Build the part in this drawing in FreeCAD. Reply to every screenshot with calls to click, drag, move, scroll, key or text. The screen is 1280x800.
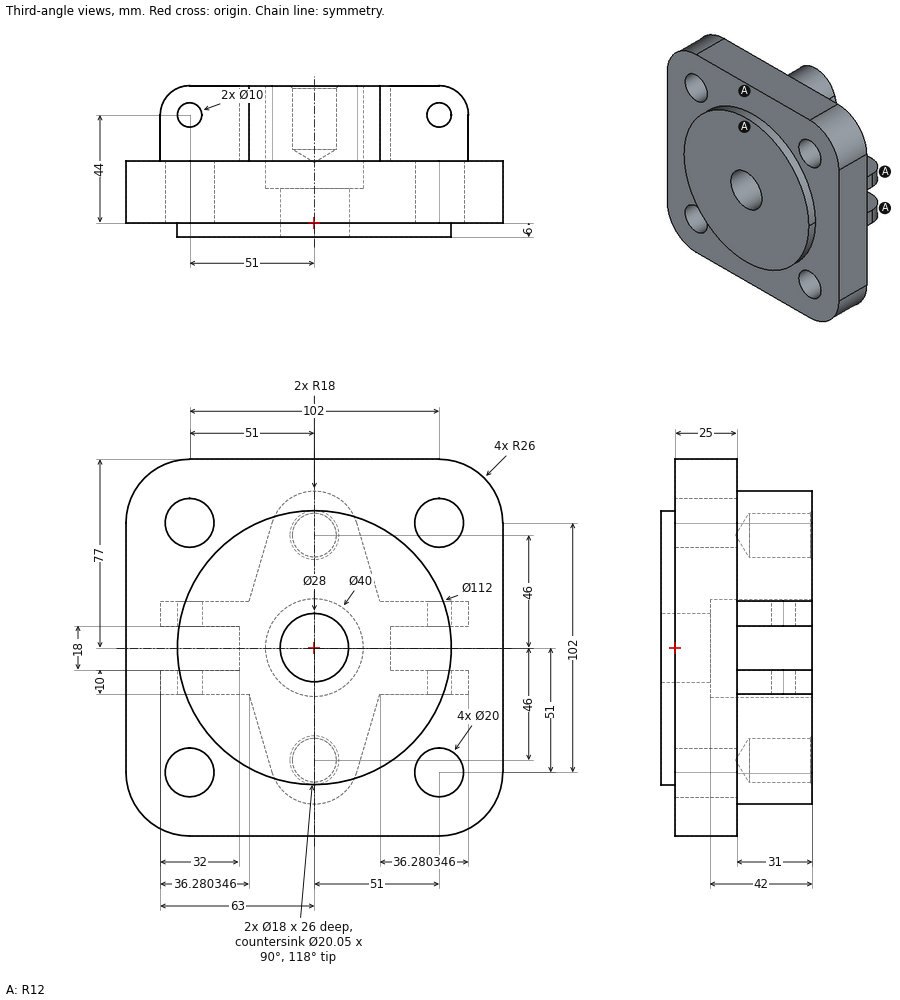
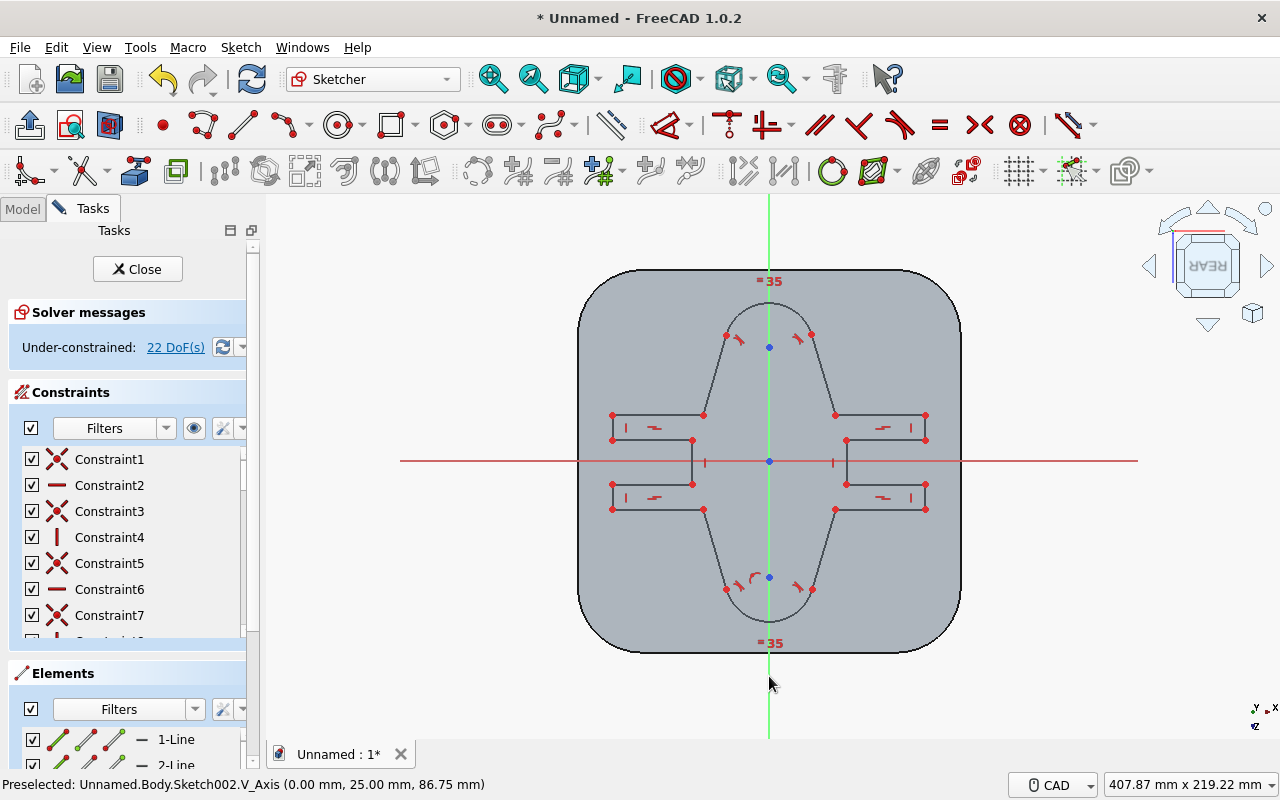
click(769, 348)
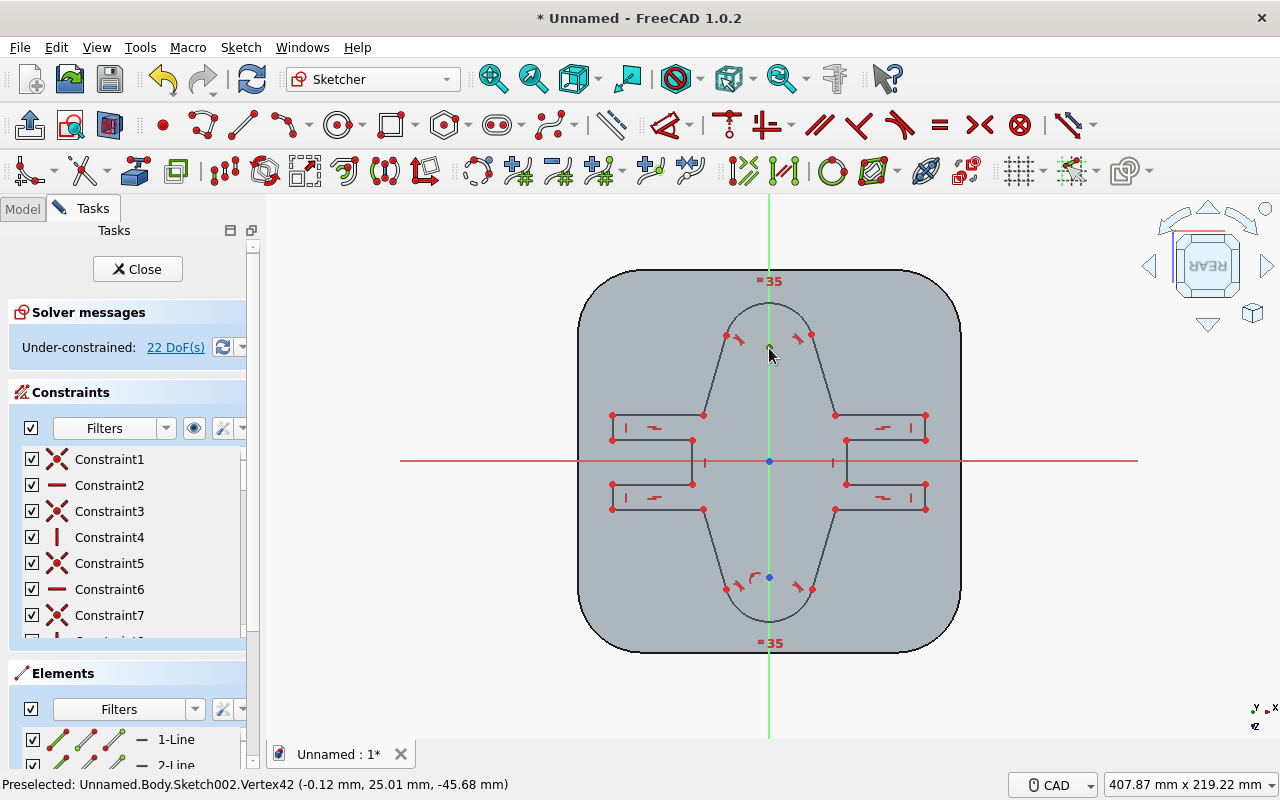
click(769, 676)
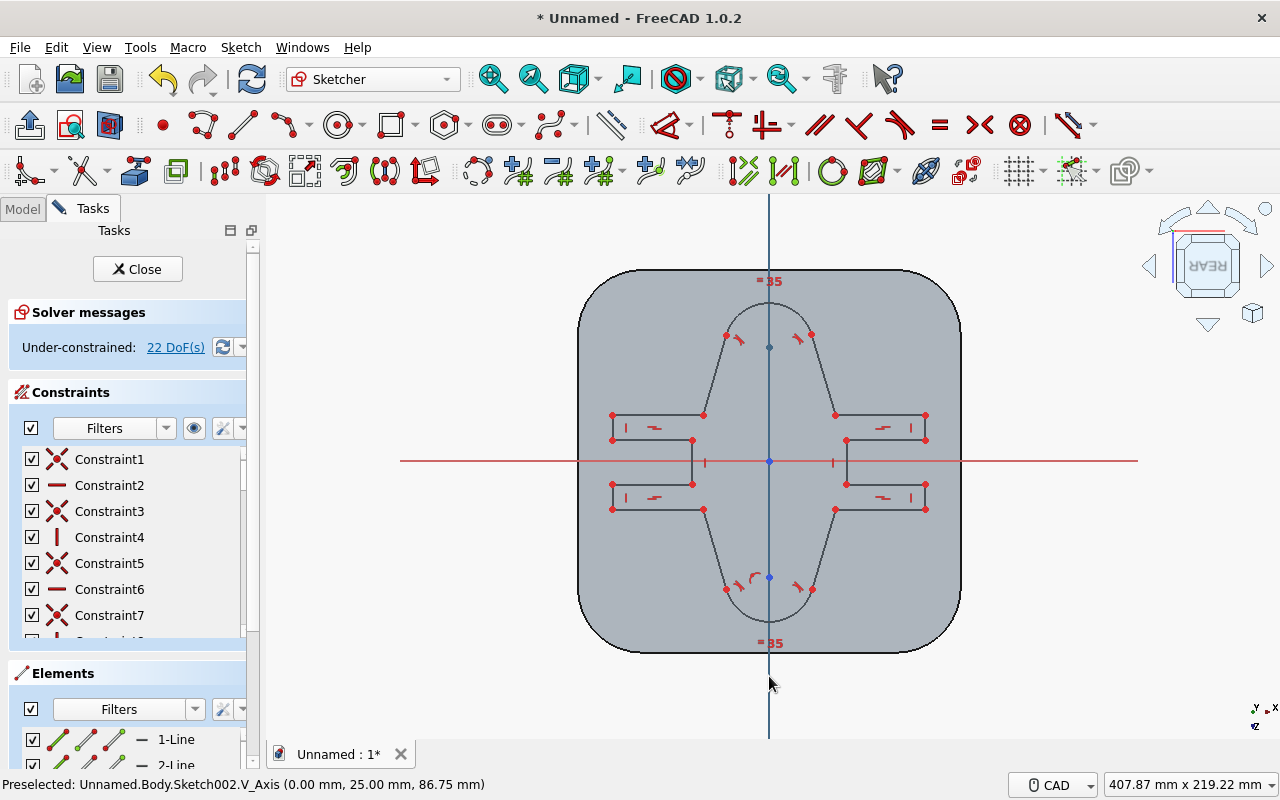
key(c)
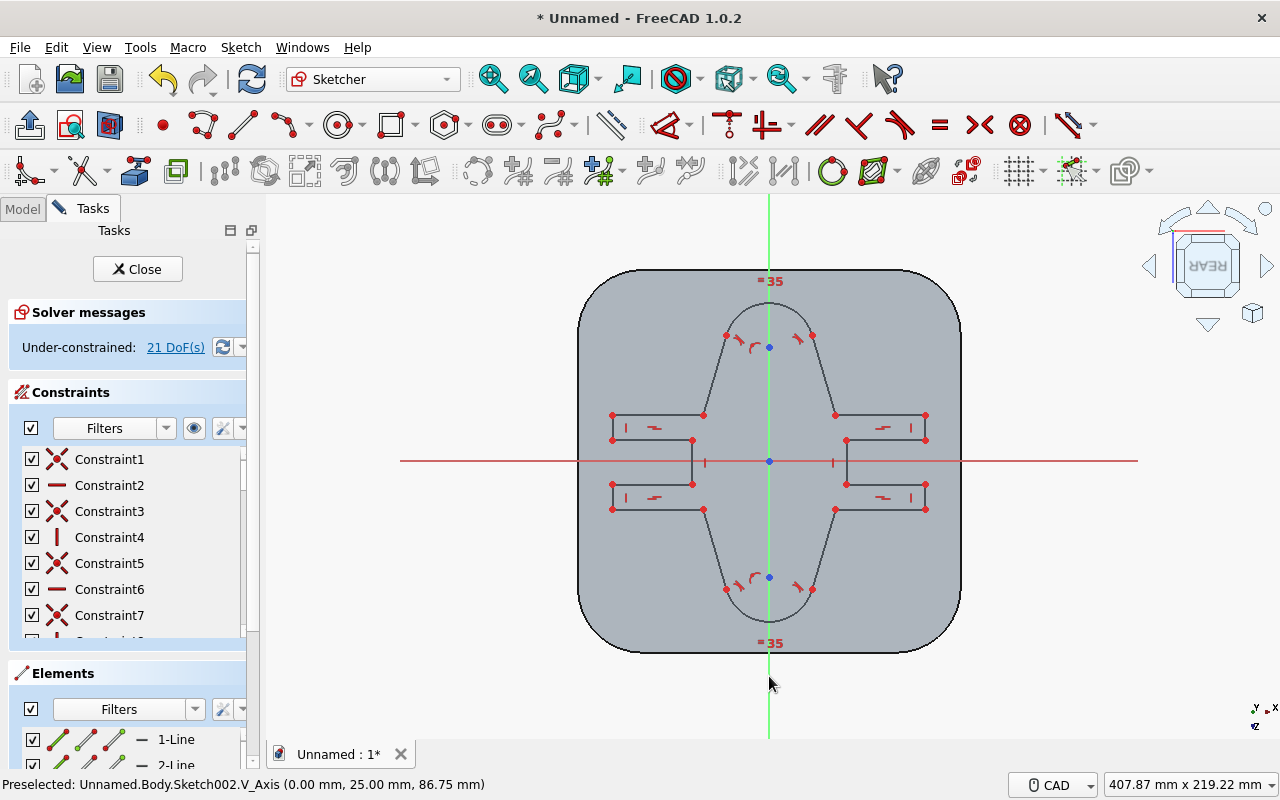
click(613, 440)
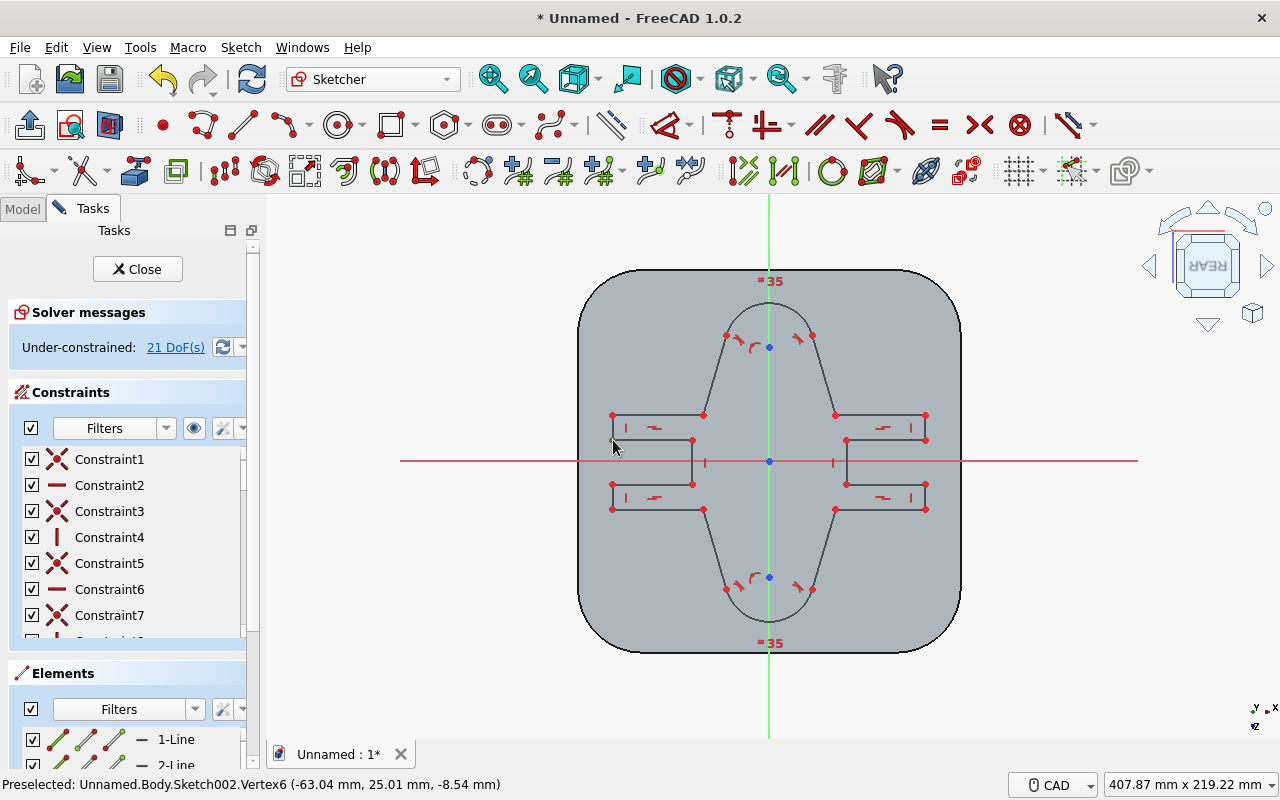
click(613, 485)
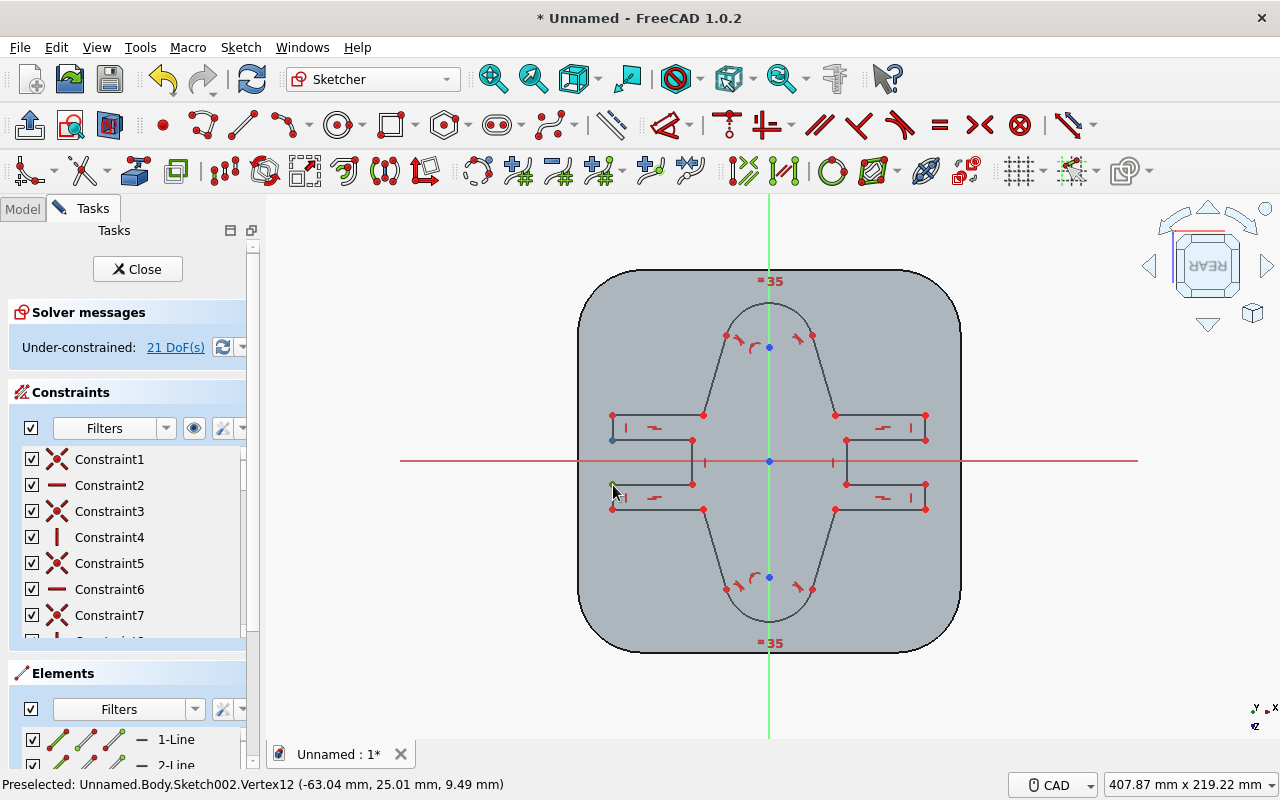
click(411, 461)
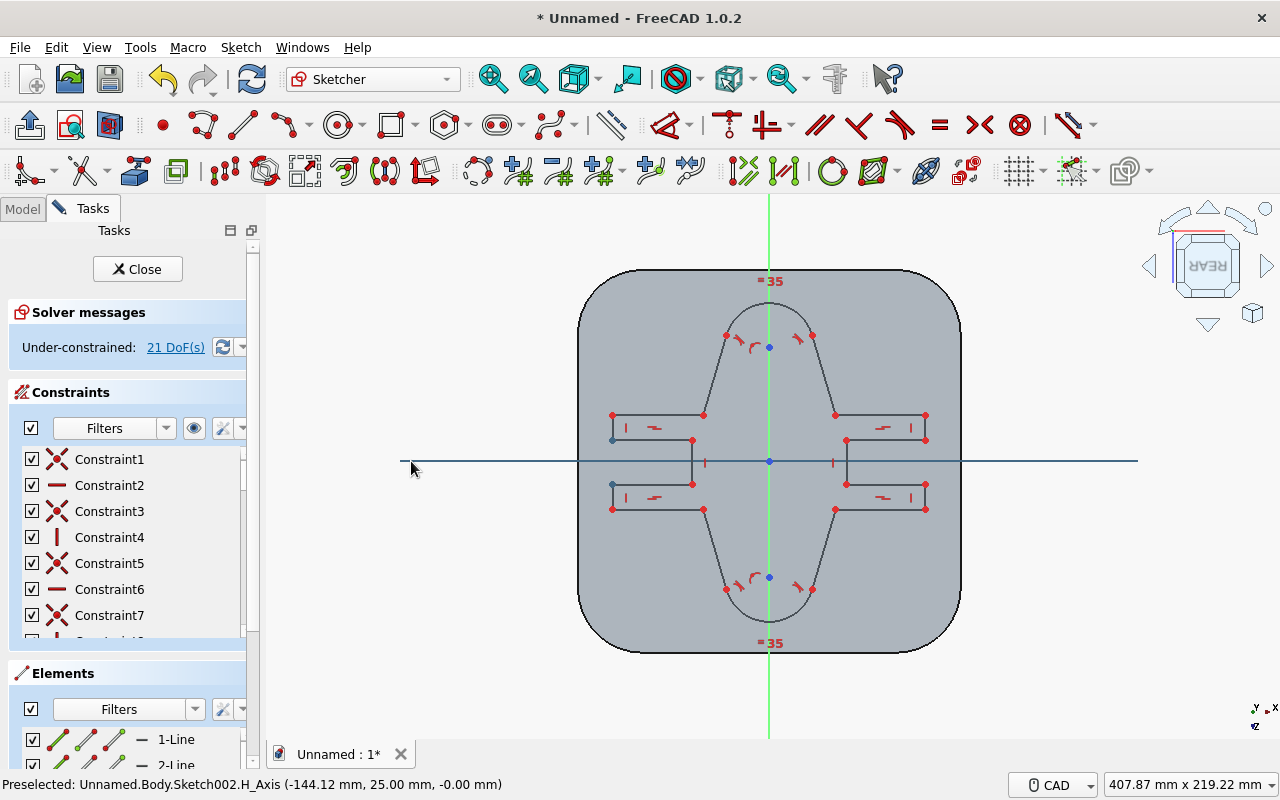
key(s)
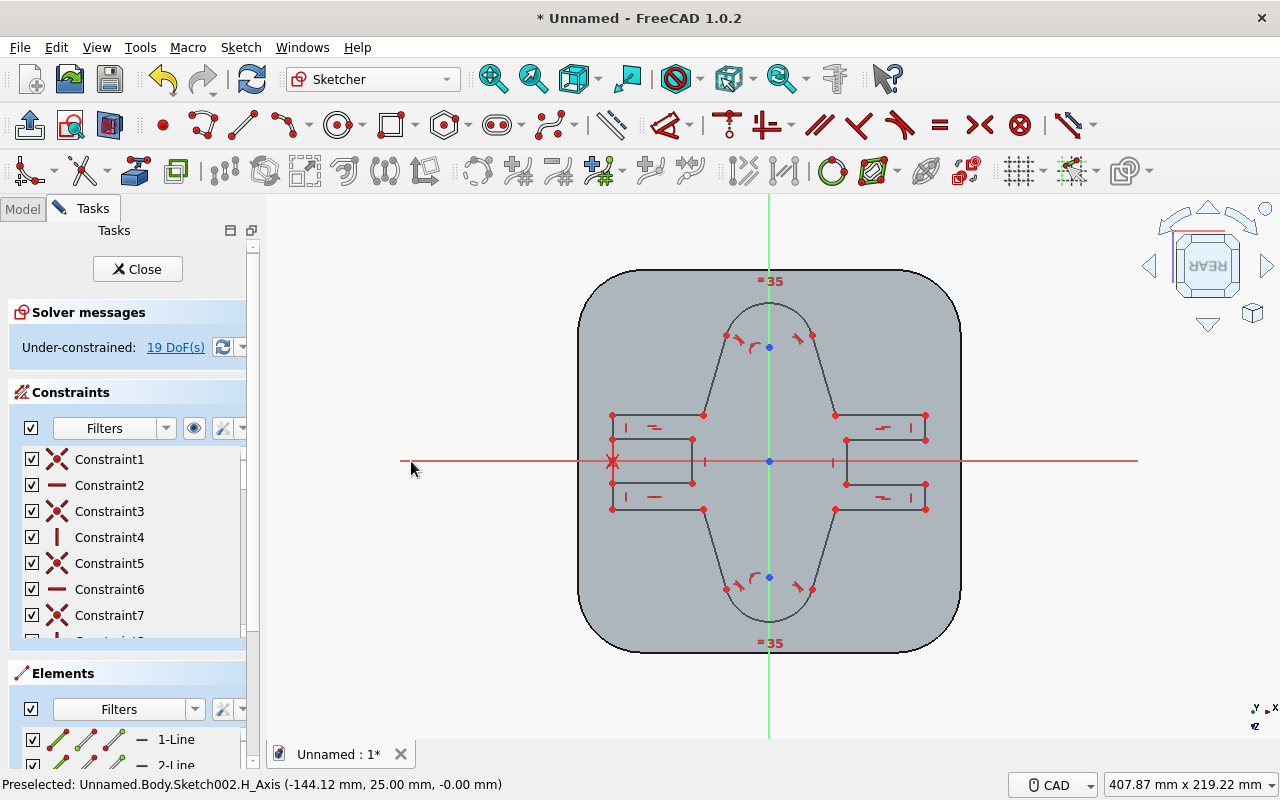
click(703, 415)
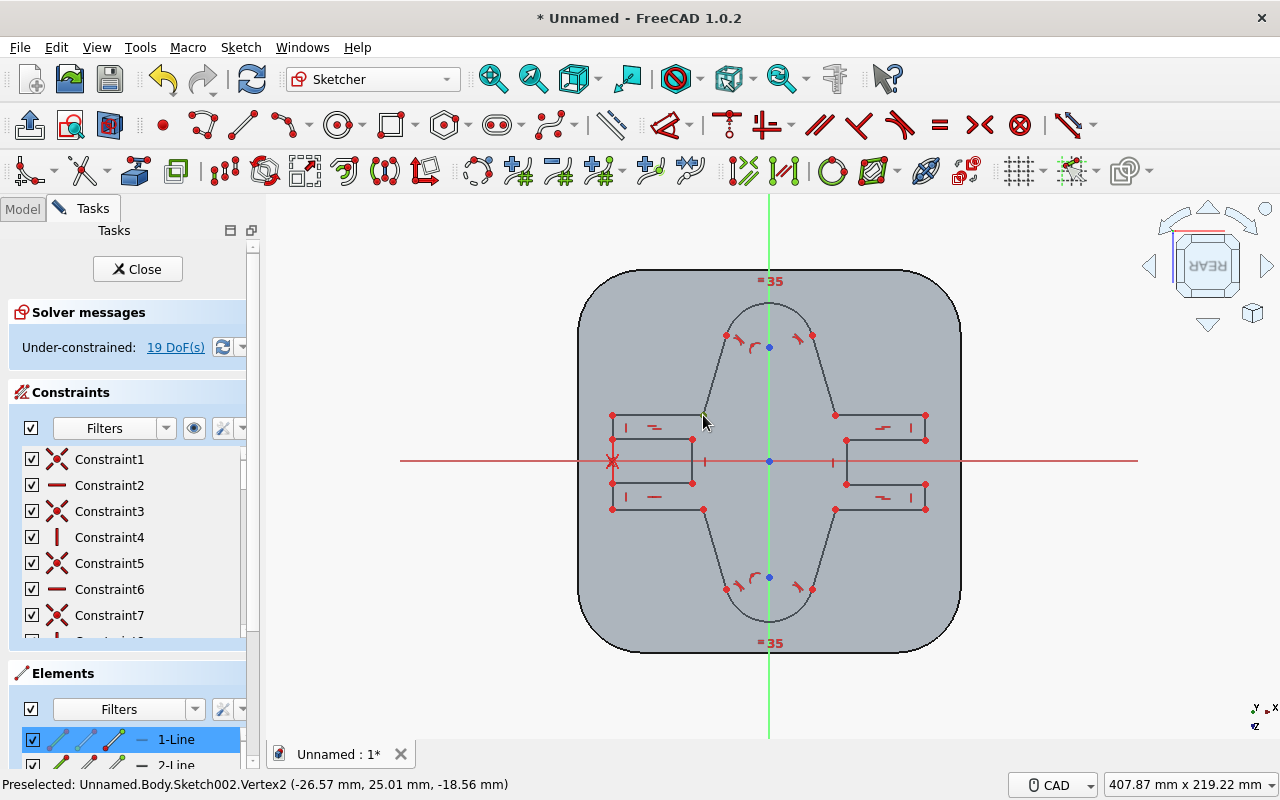
click(703, 510)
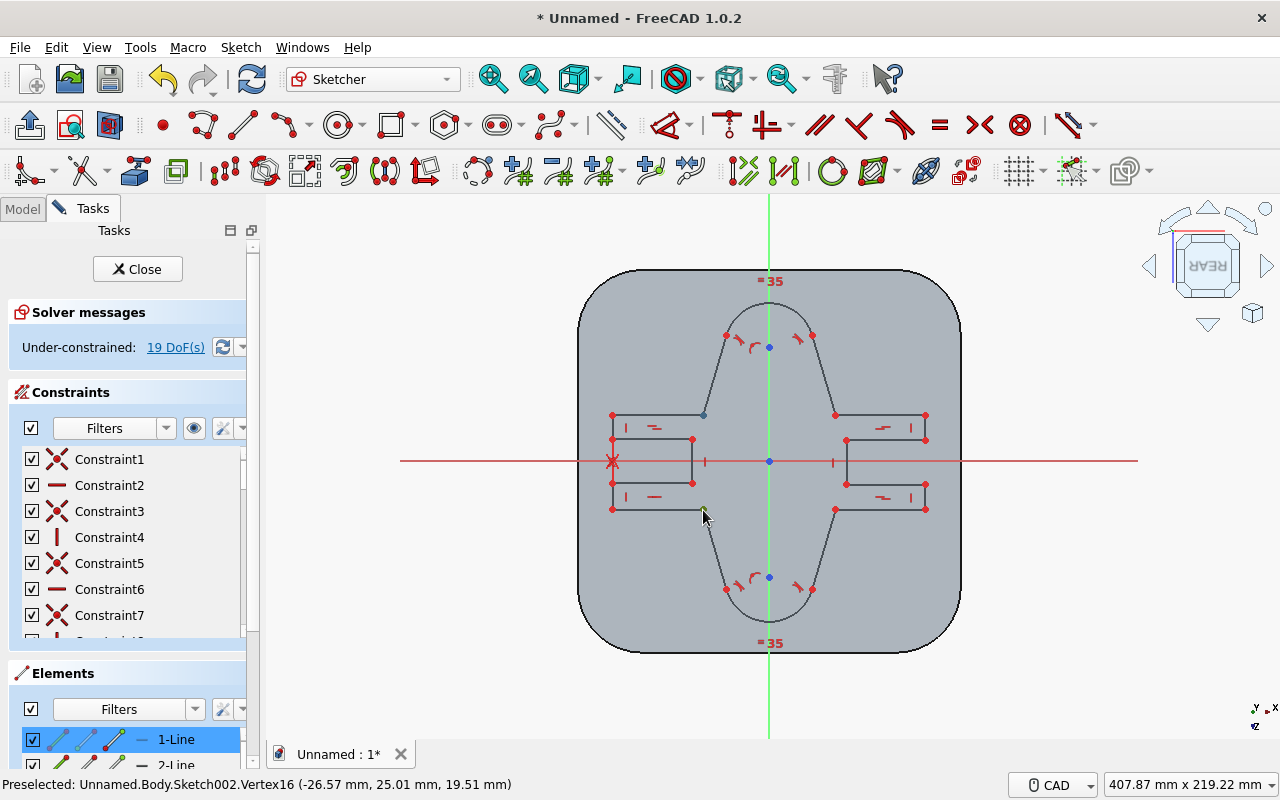
click(411, 461)